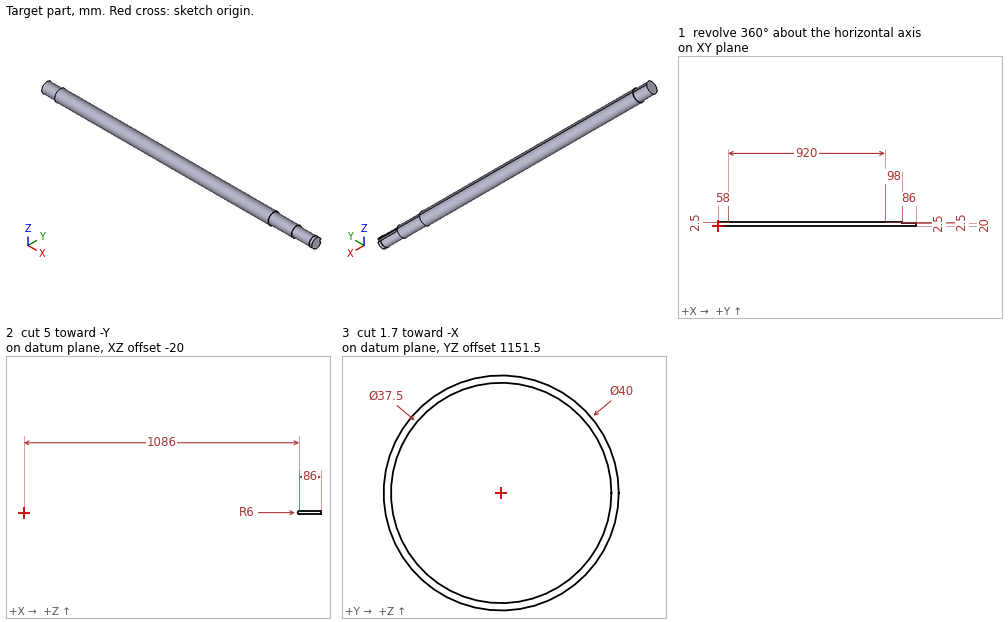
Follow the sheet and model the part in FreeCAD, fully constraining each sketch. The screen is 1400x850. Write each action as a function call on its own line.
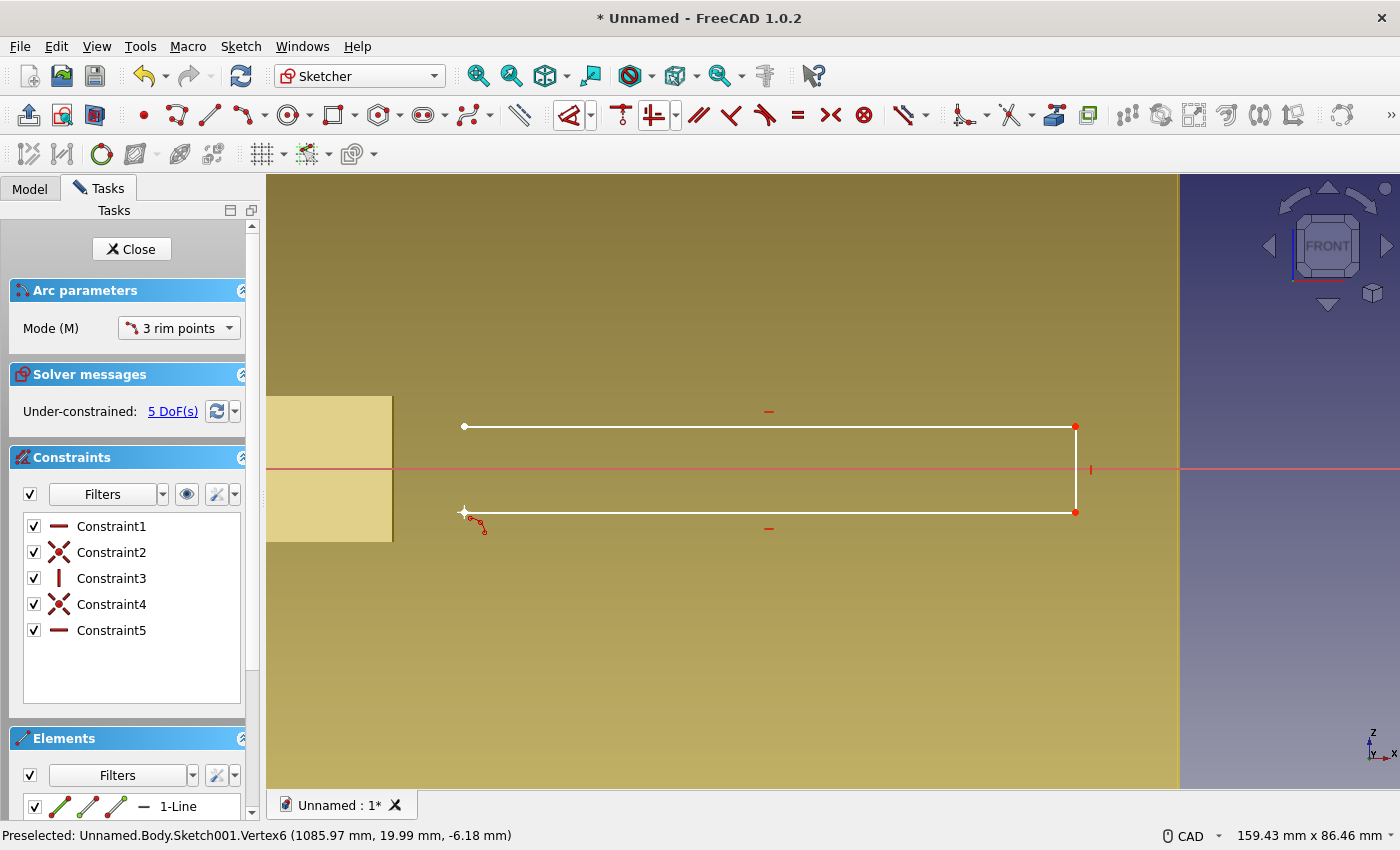
click(464, 513)
click(464, 427)
click(430, 444)
key(Escape)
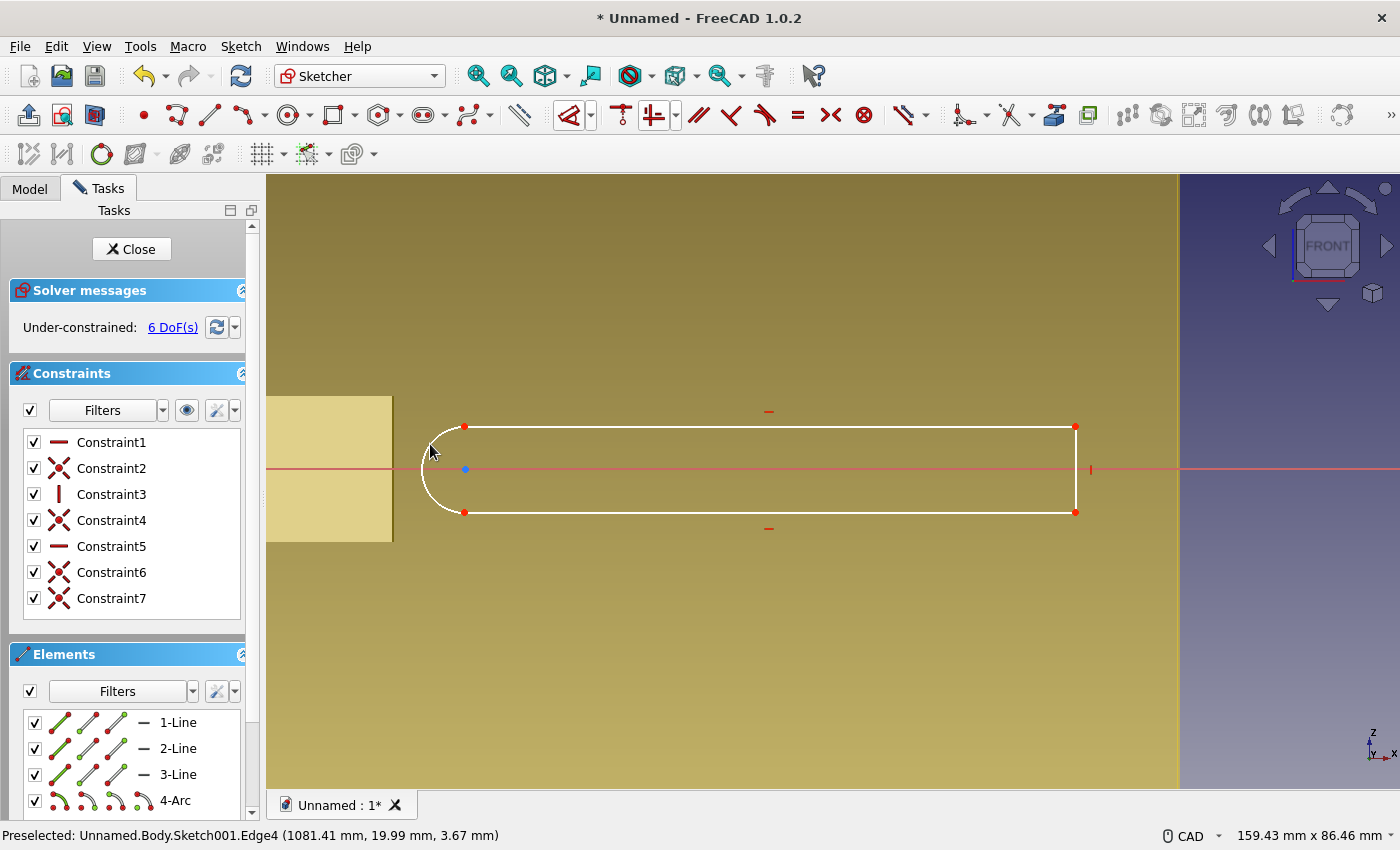
click(648, 427)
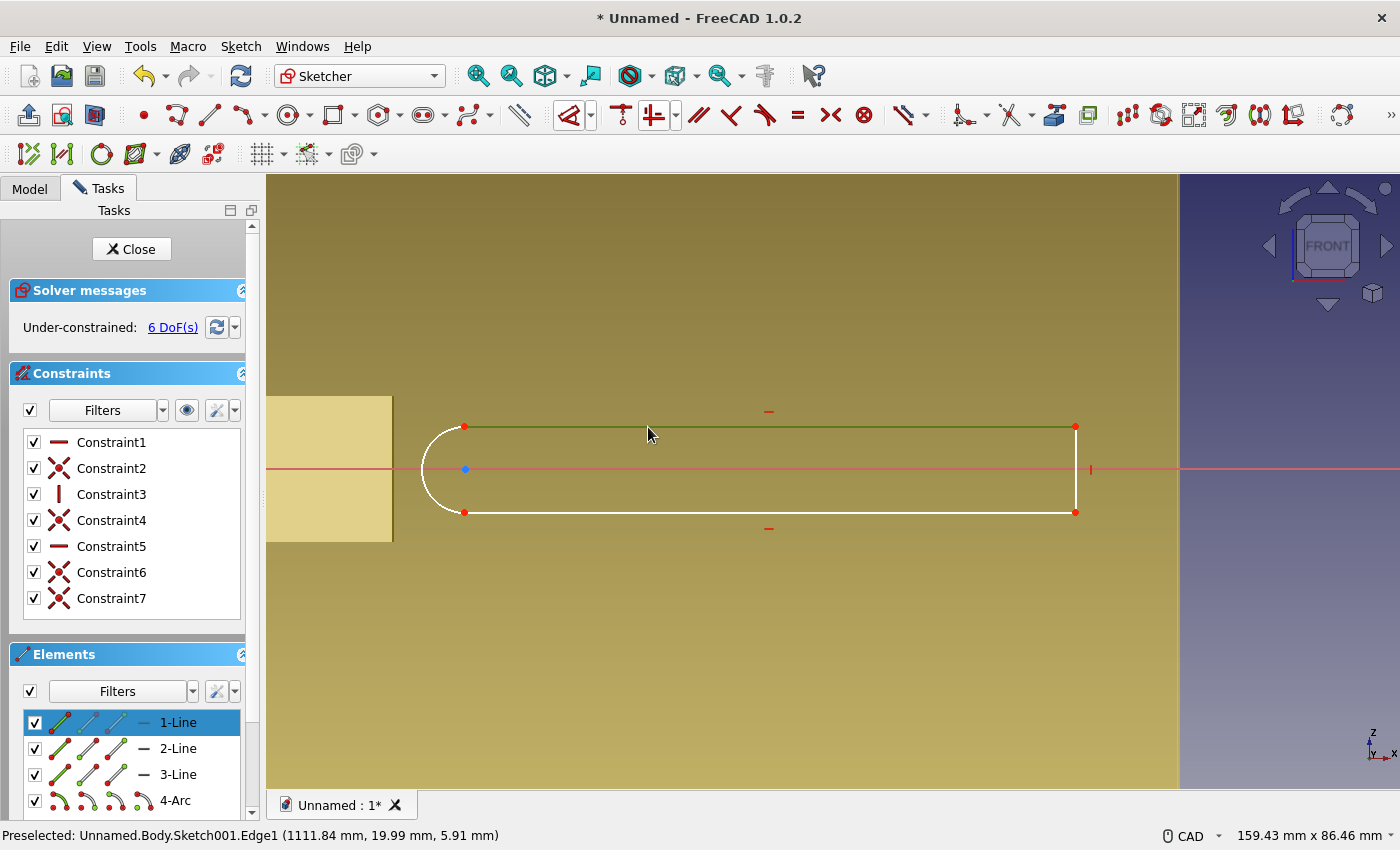
click(430, 445)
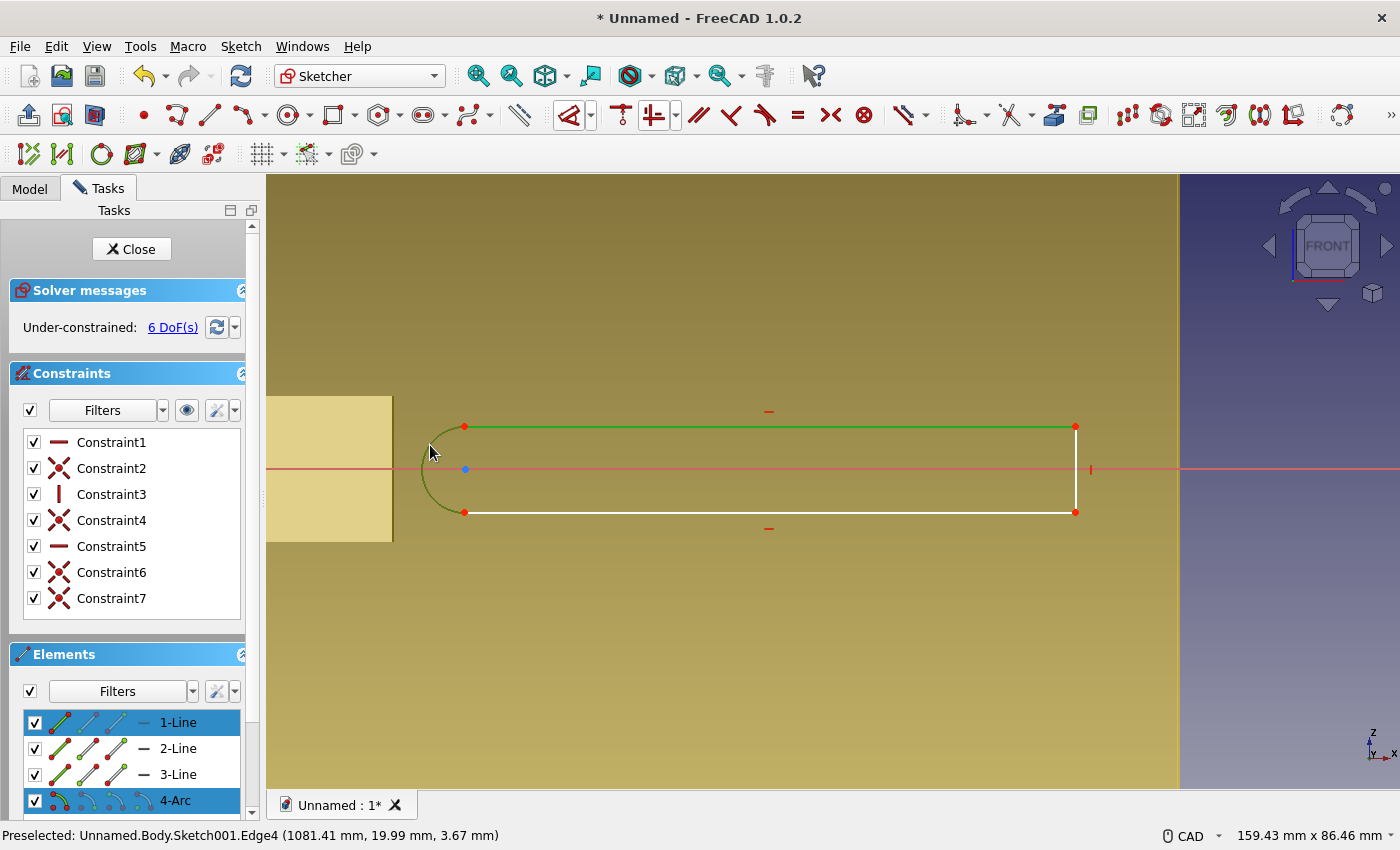
click(765, 116)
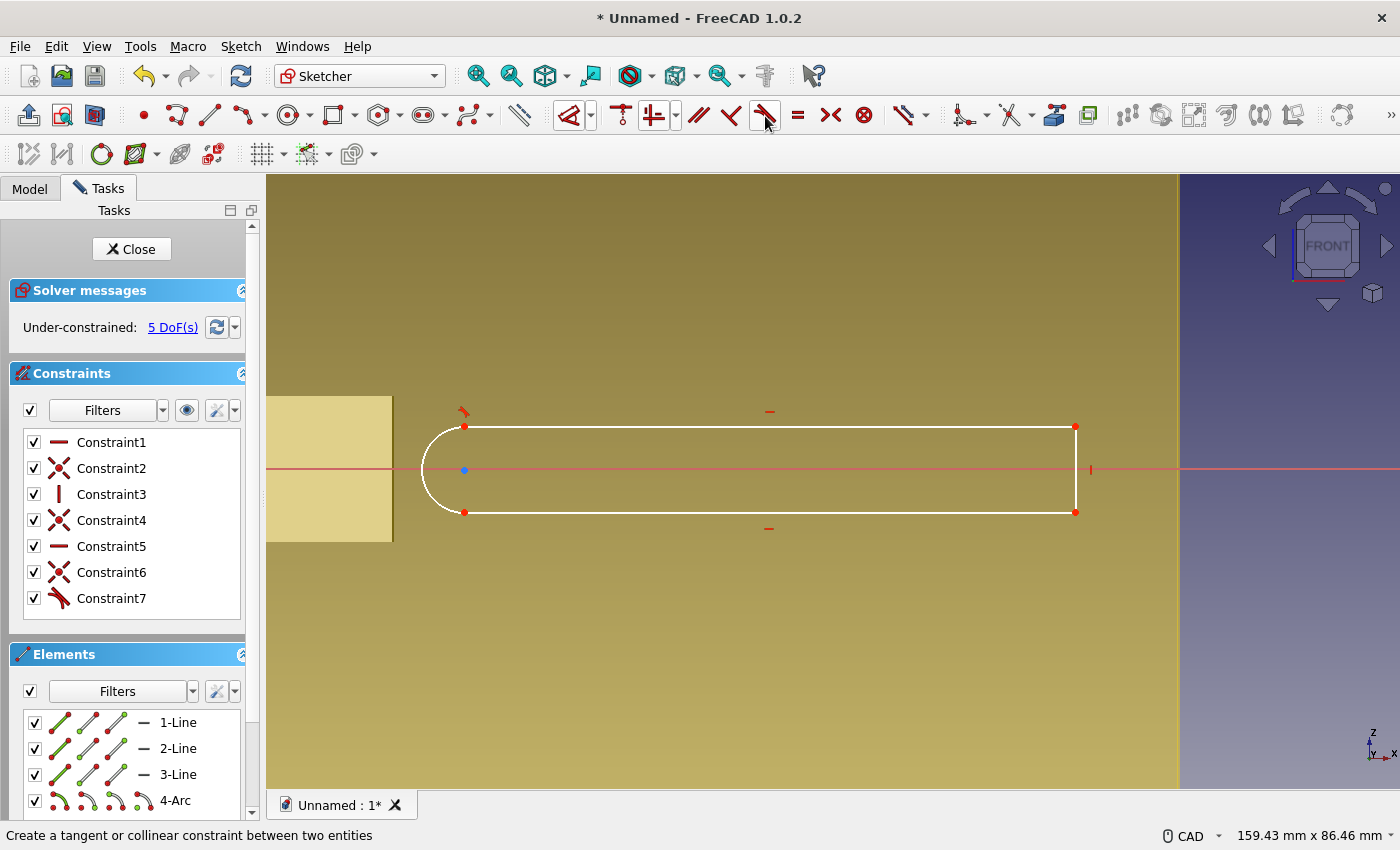
click(892, 513)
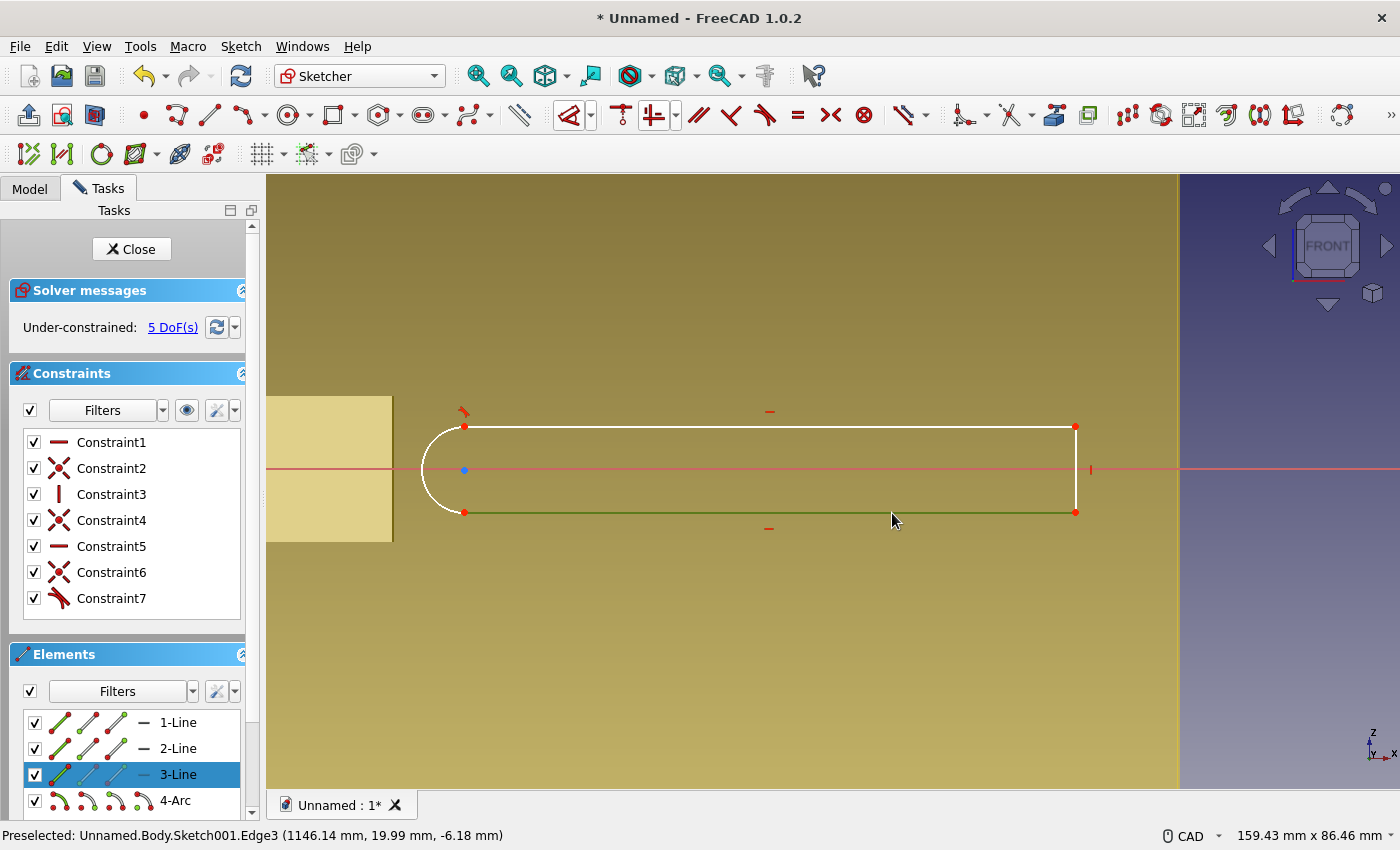
click(430, 444)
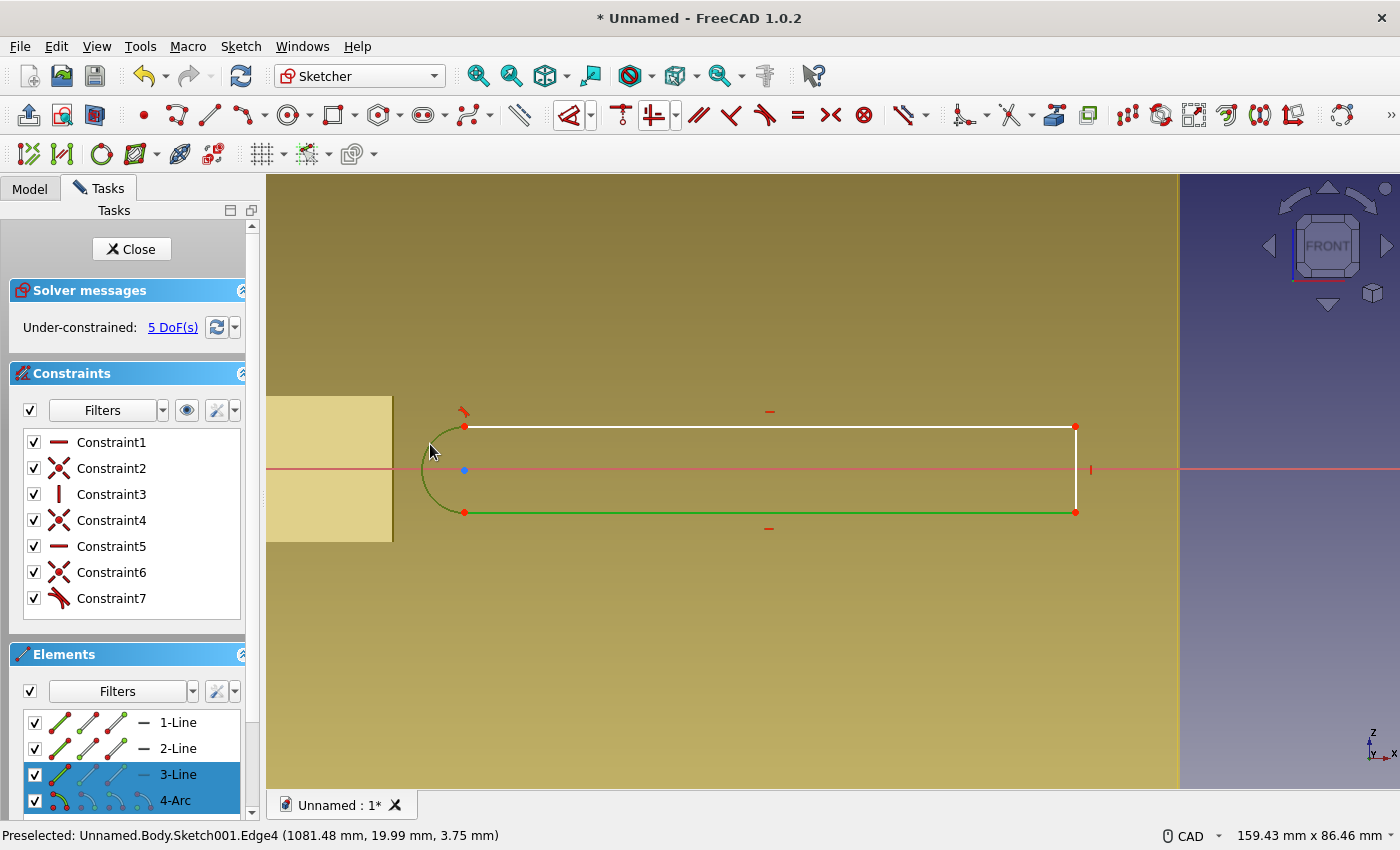
click(765, 116)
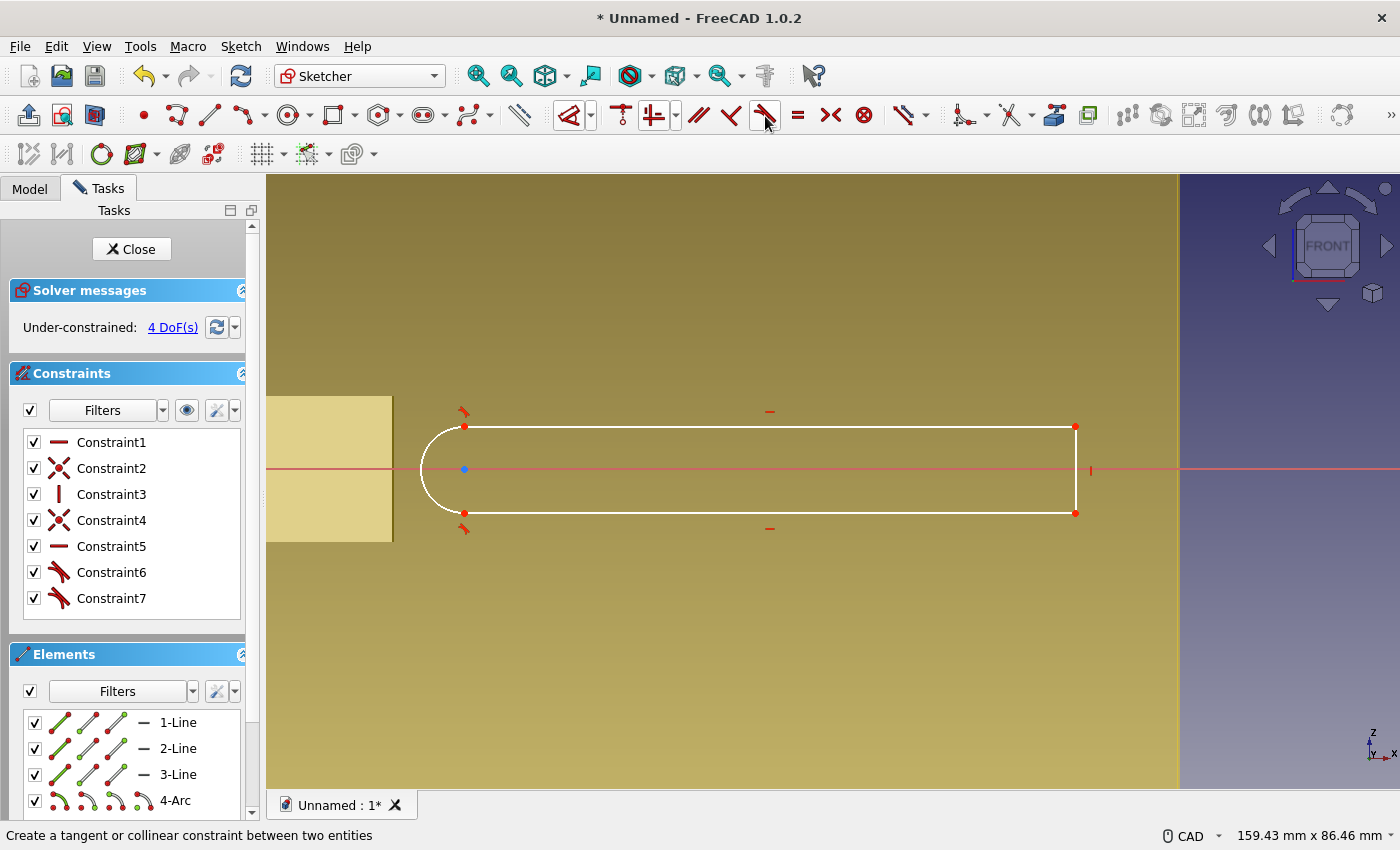
click(464, 470)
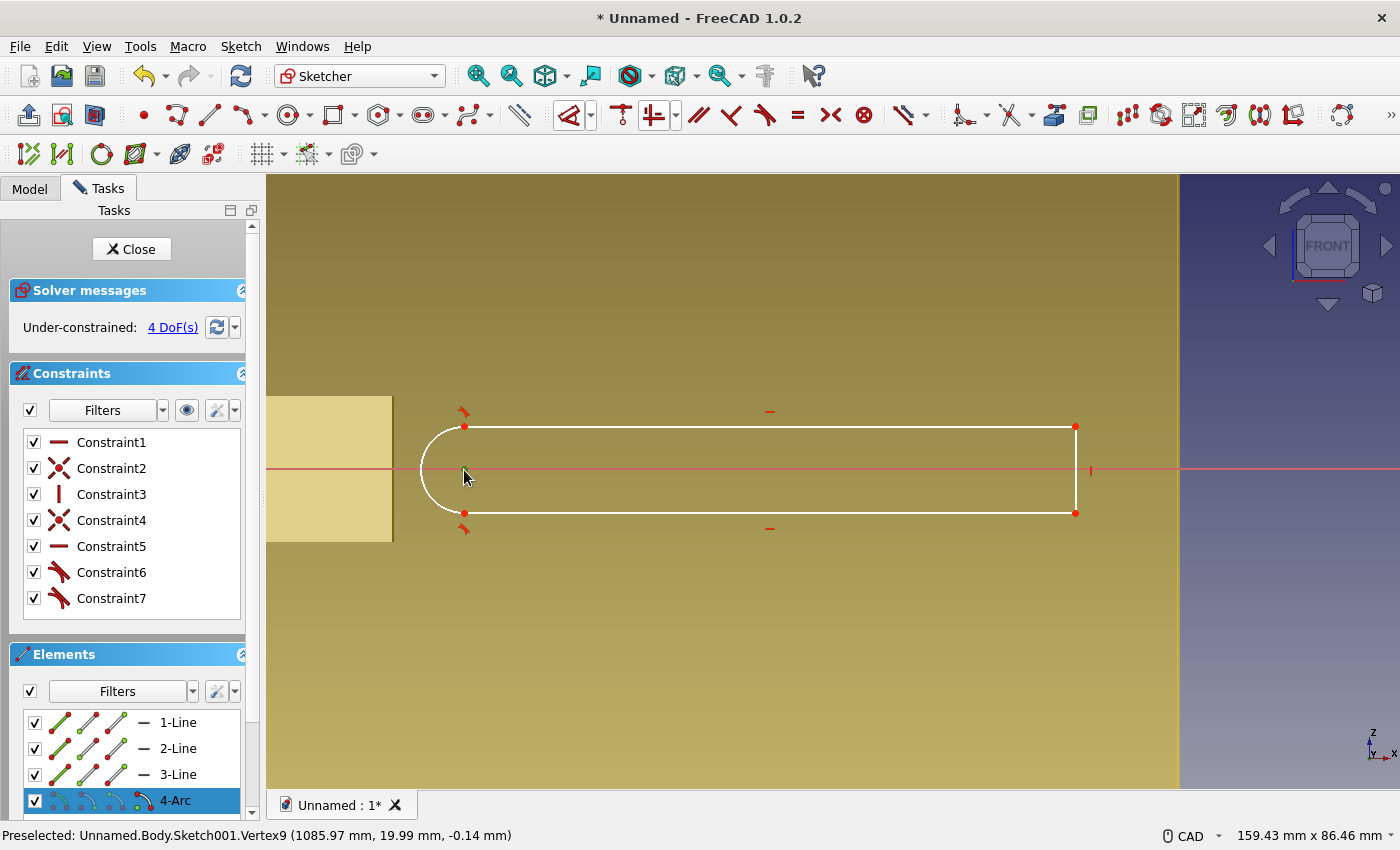
click(361, 469)